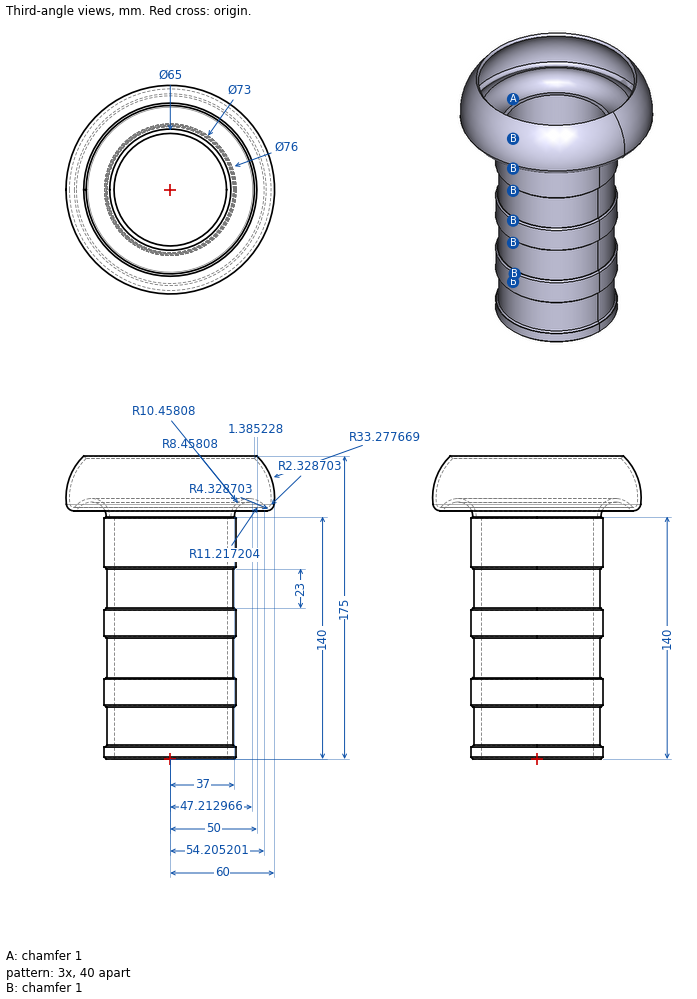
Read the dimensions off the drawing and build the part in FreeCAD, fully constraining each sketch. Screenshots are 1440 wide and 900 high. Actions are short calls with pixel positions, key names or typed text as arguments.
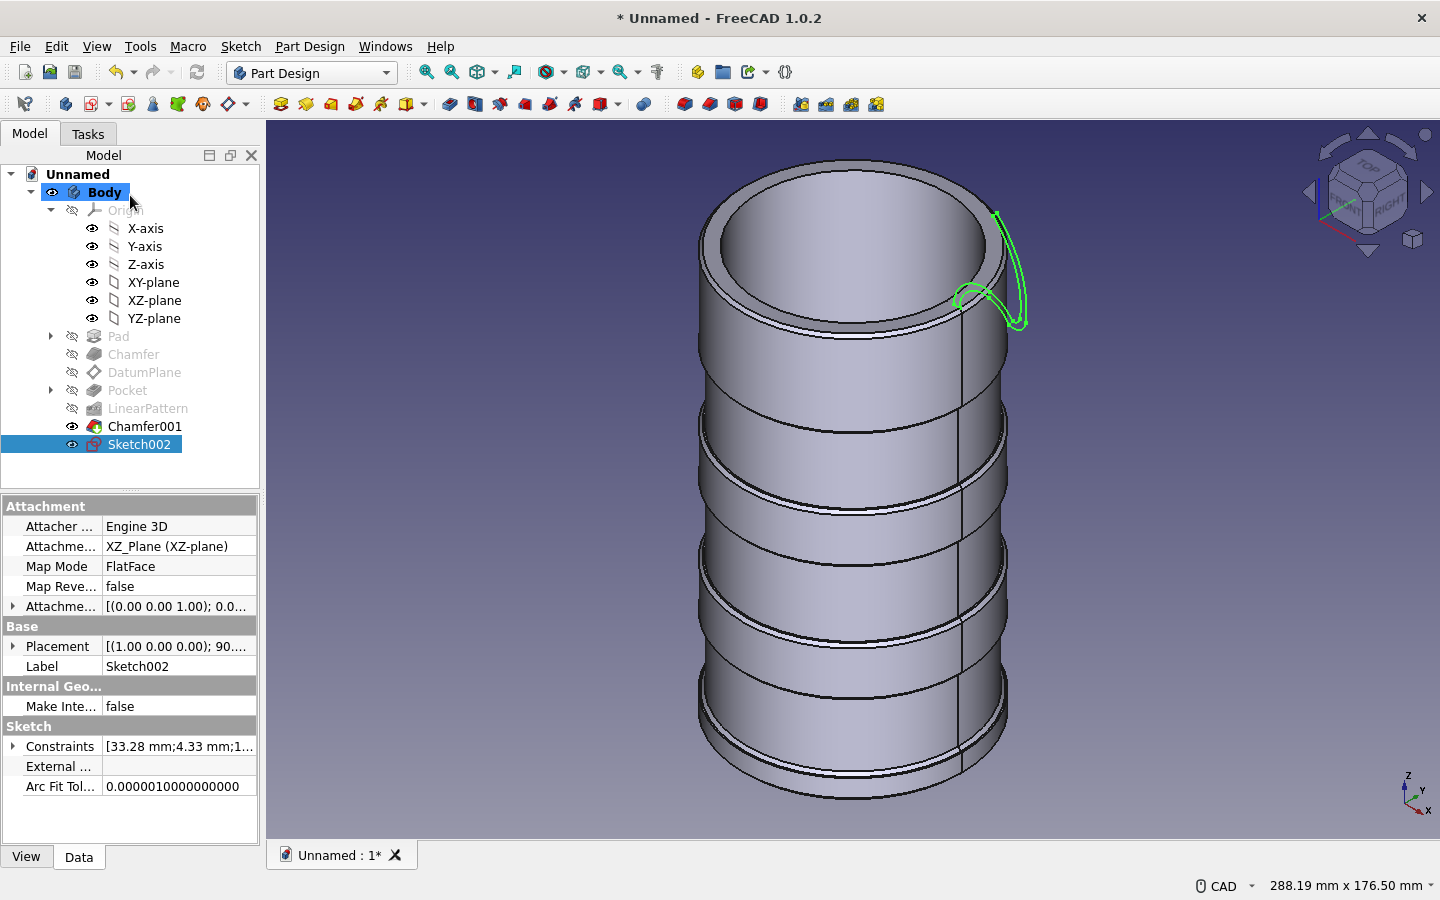
click(306, 104)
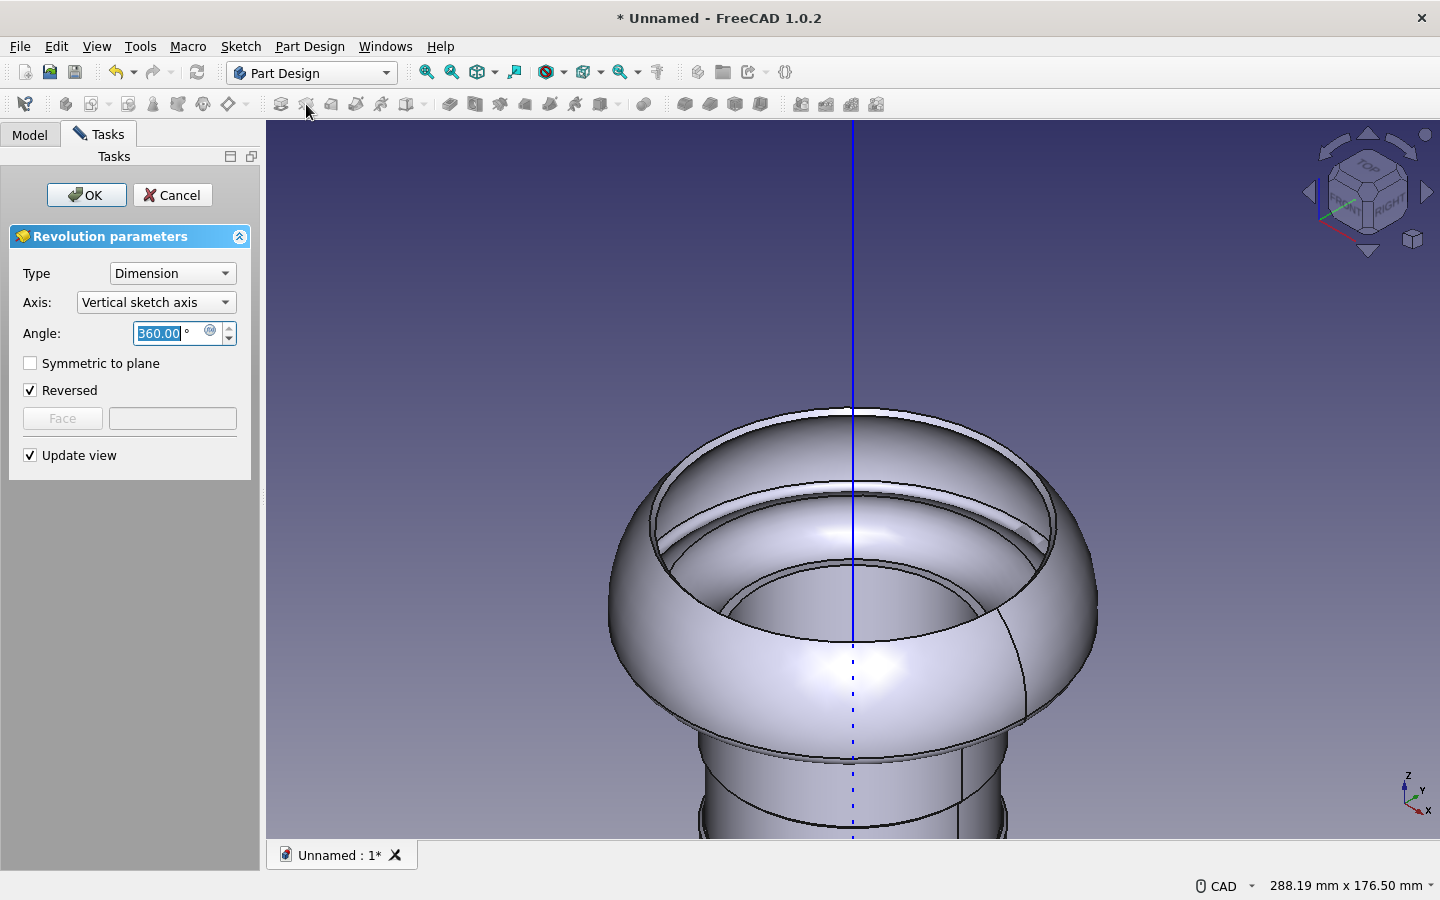
click(87, 195)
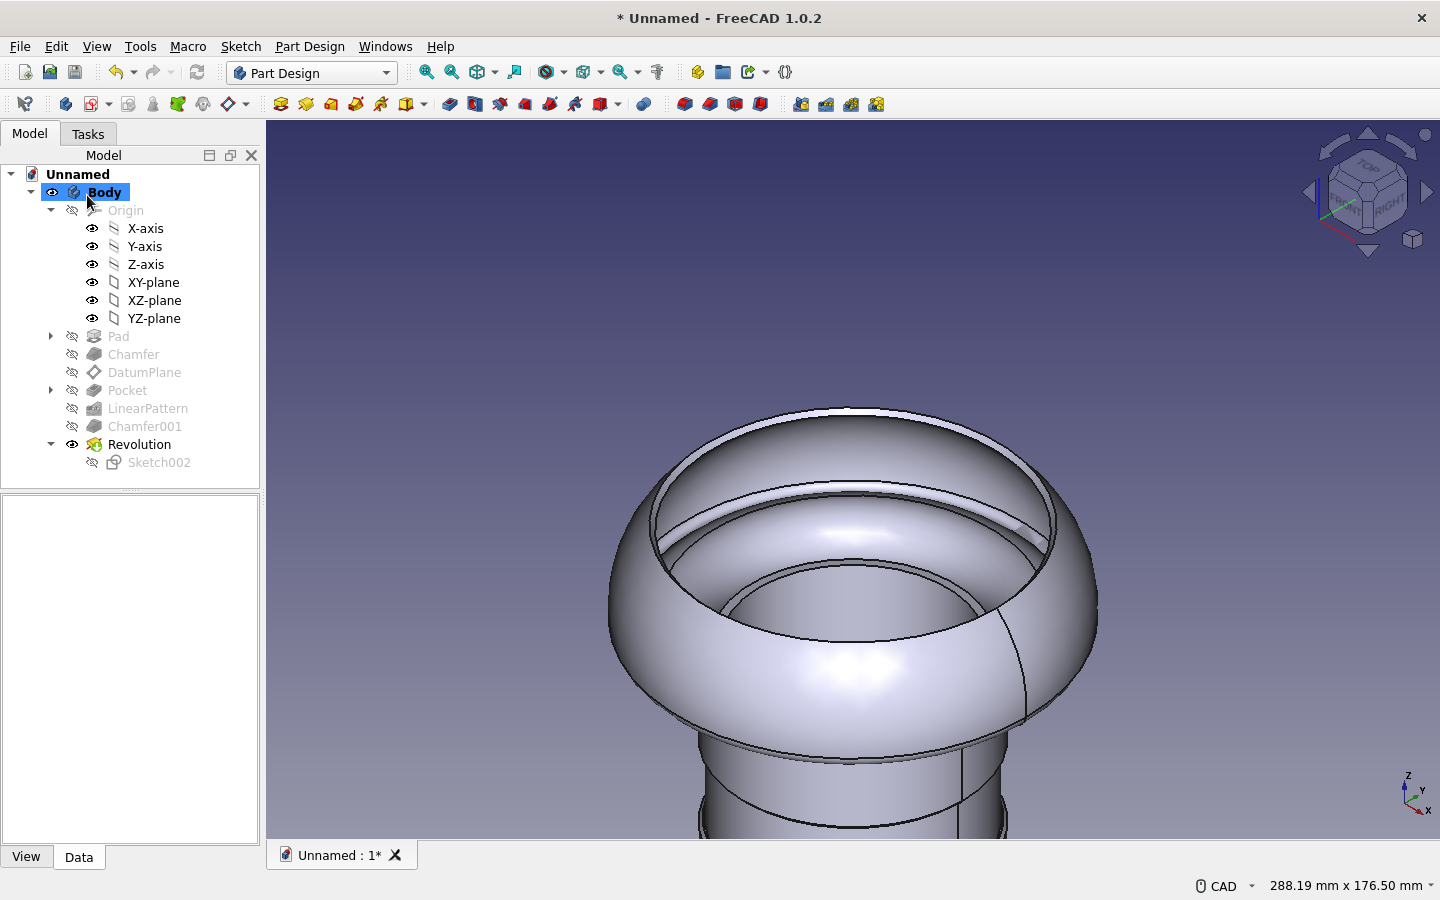
click(427, 72)